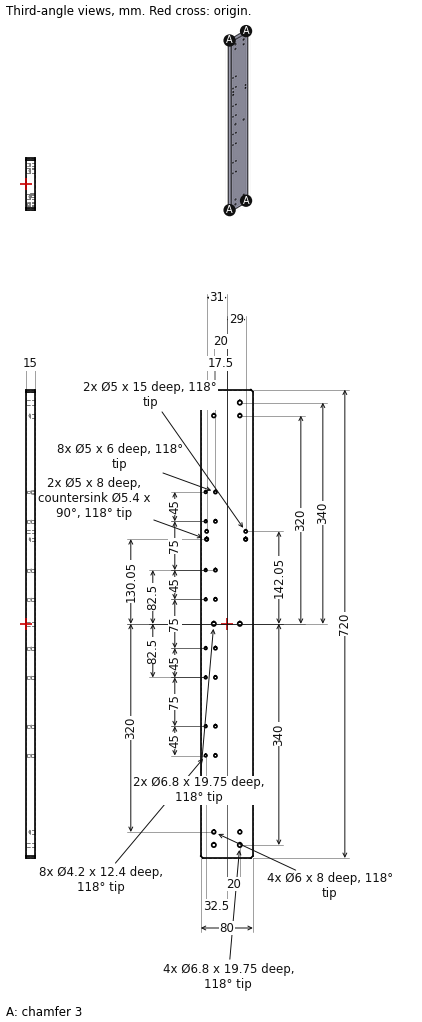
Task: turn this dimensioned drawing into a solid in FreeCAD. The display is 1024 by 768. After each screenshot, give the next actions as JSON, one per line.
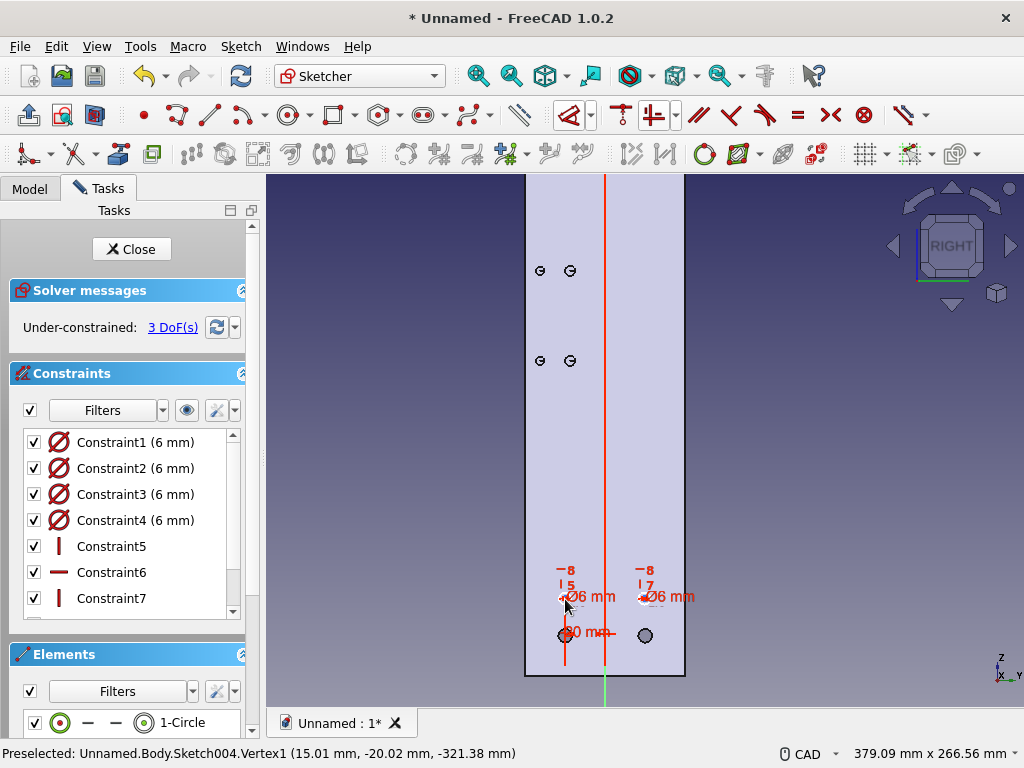
{"action": "scroll", "coordinate": [567, 599], "scroll_direction": "down", "scroll_amount": 7}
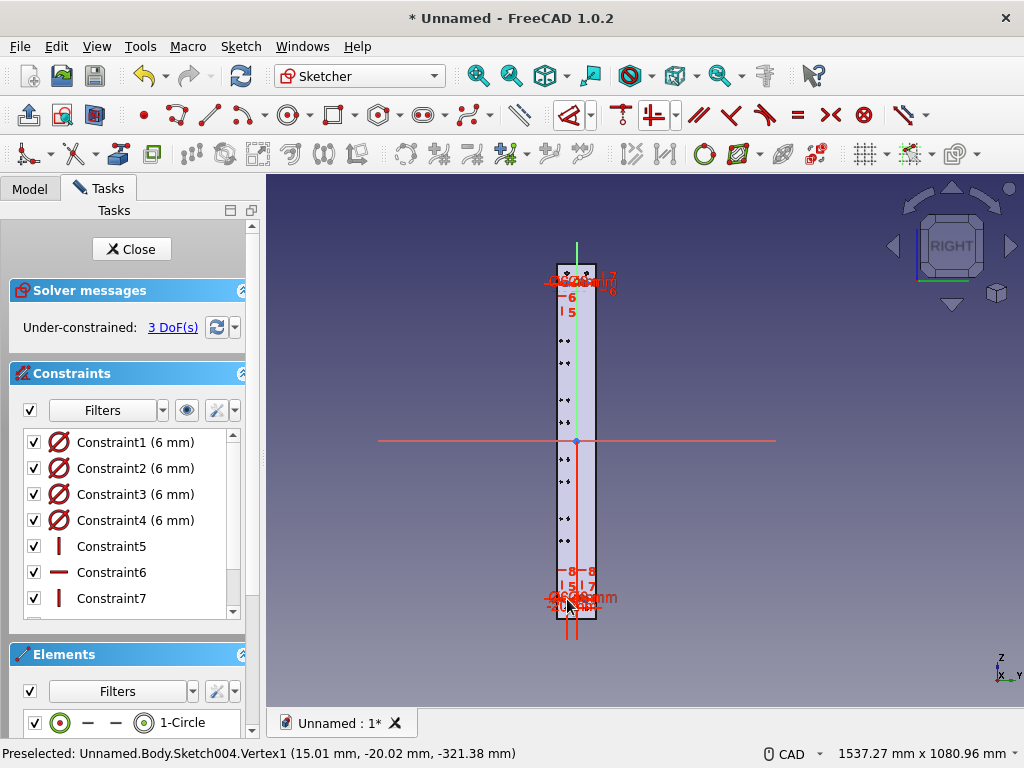
{"action": "scroll", "coordinate": [586, 284], "scroll_direction": "up", "scroll_amount": 7}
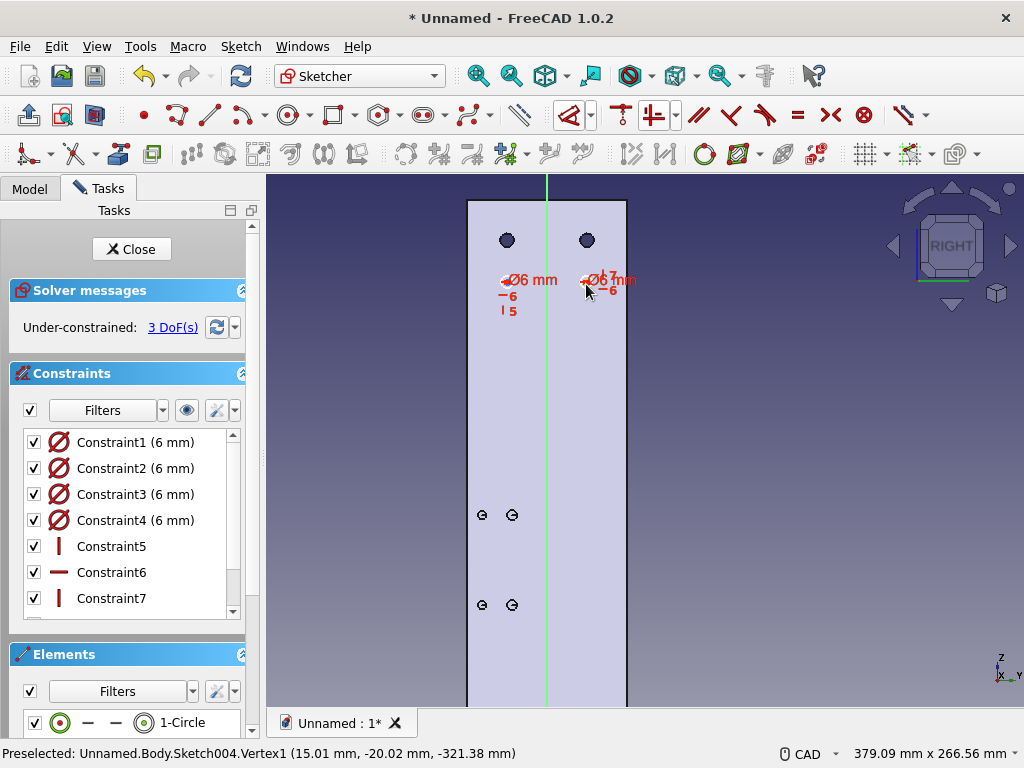
{"action": "left_click", "coordinate": [586, 282]}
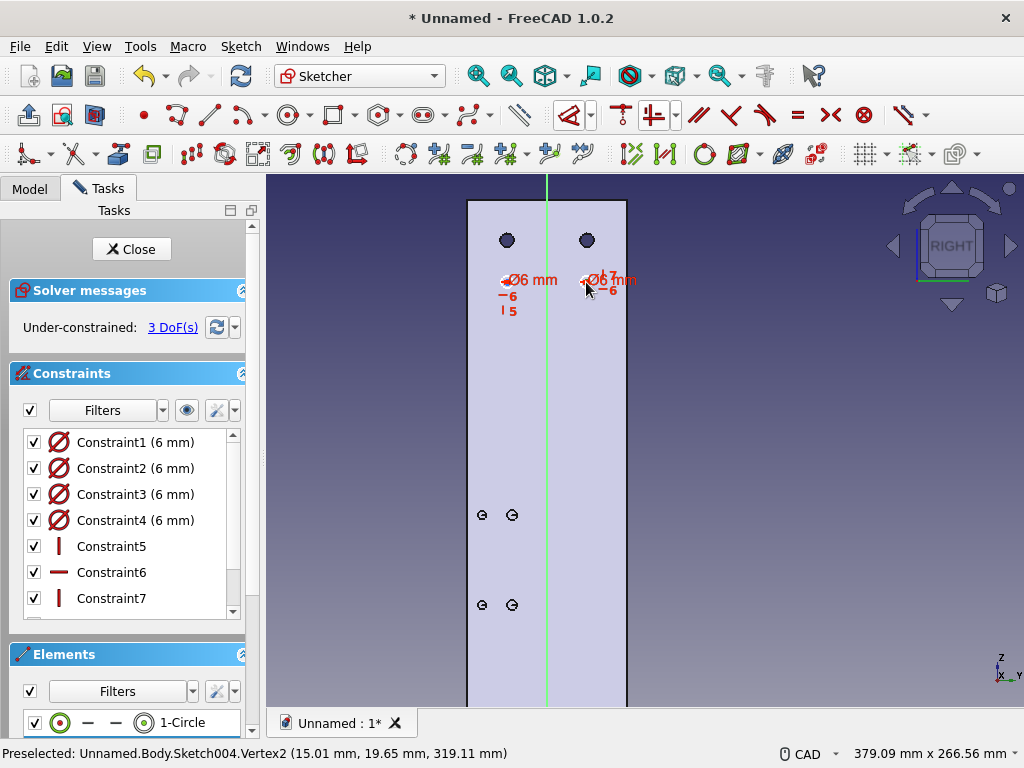
{"action": "left_click", "coordinate": [590, 116]}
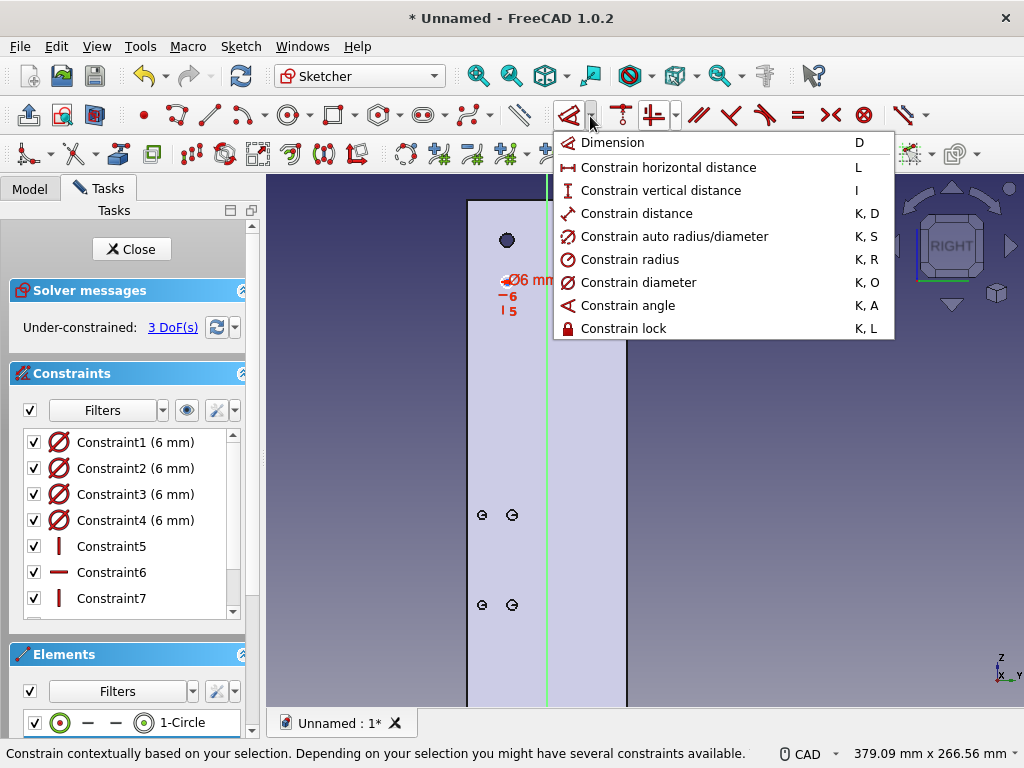
{"action": "left_click", "coordinate": [724, 168]}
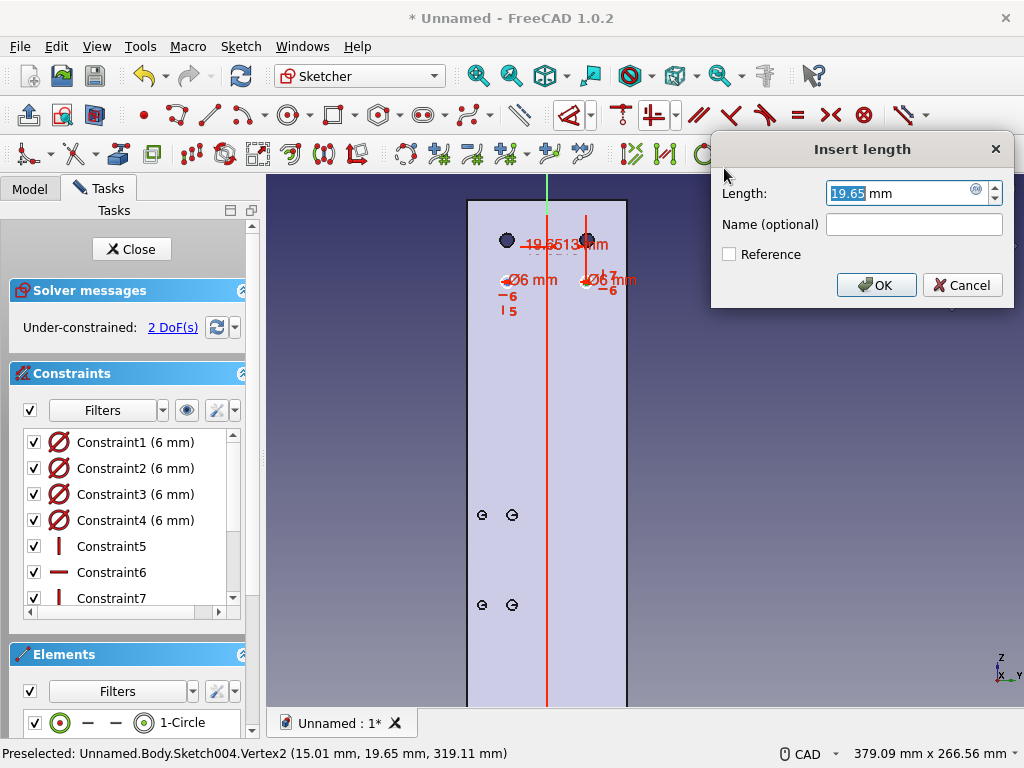
{"action": "type", "text": "20"}
{"action": "key", "text": "Return"}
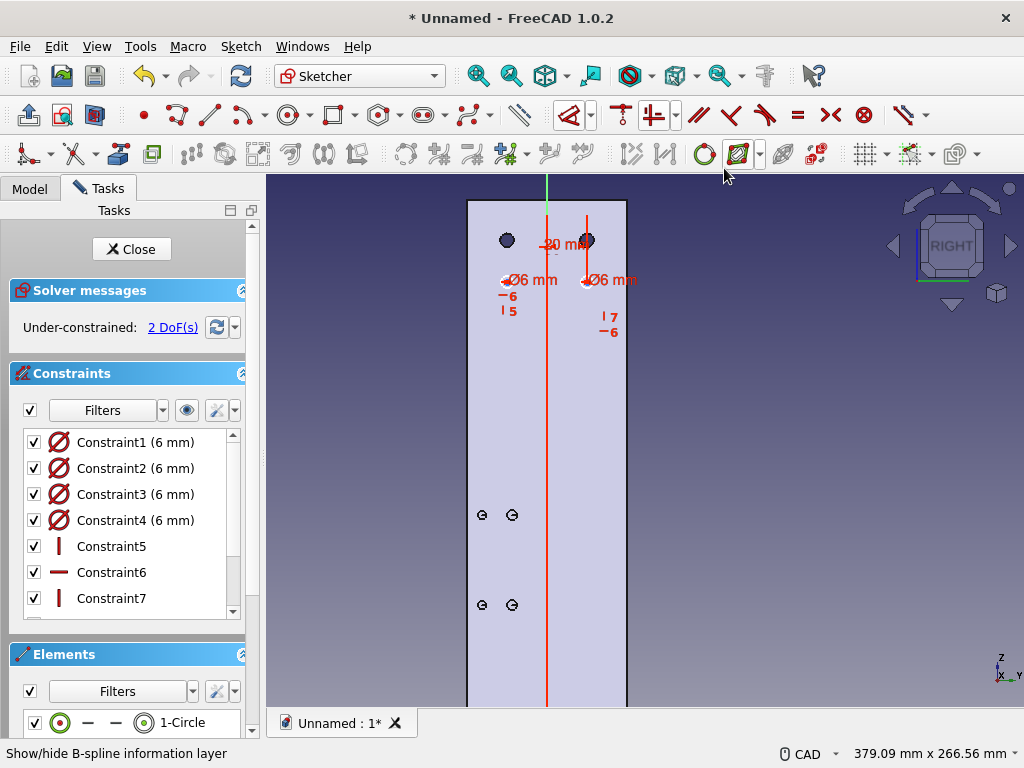
{"action": "scroll", "coordinate": [586, 284], "scroll_direction": "down", "scroll_amount": 7}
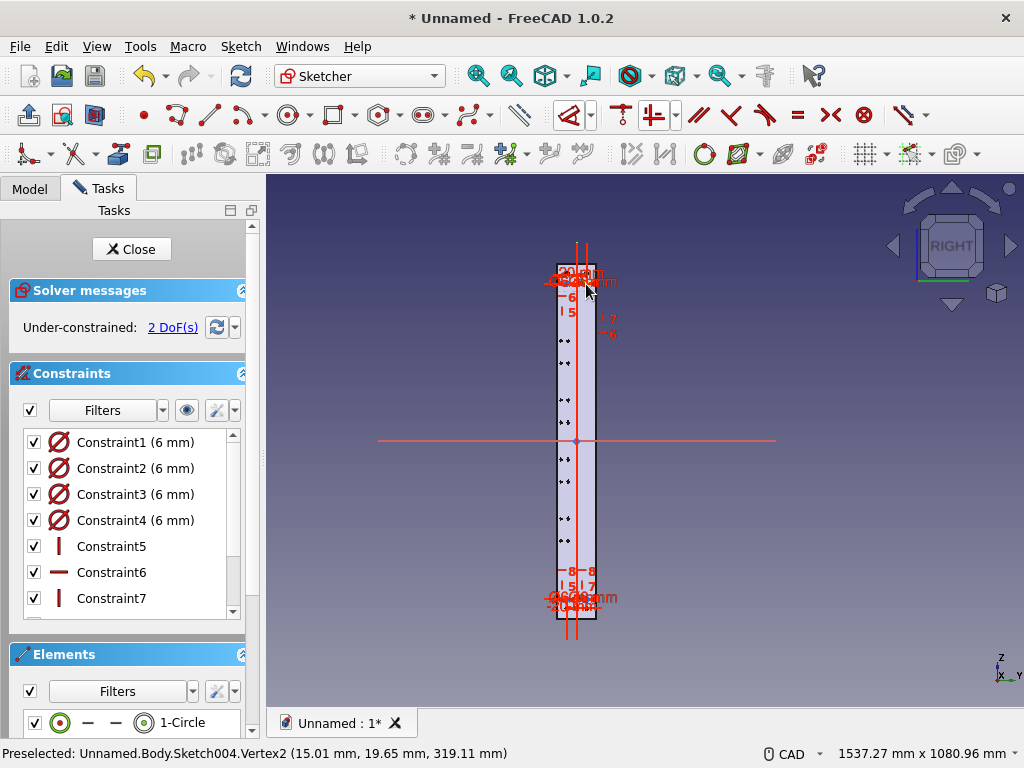
{"action": "left_click", "coordinate": [567, 599]}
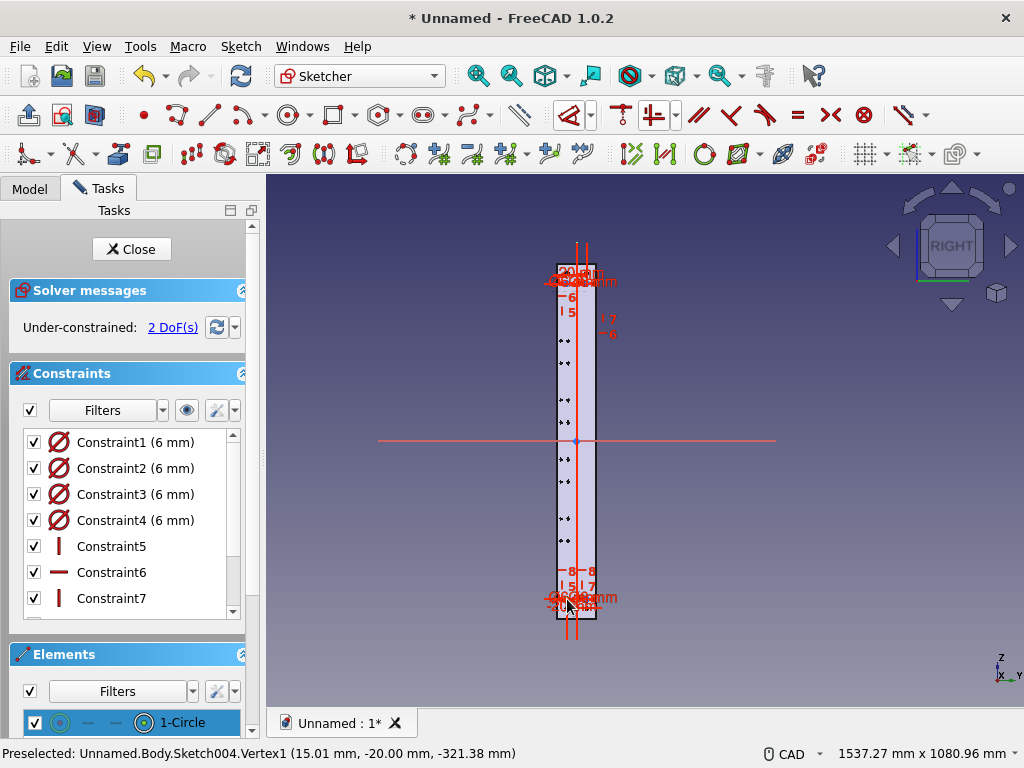
{"action": "left_click", "coordinate": [590, 116]}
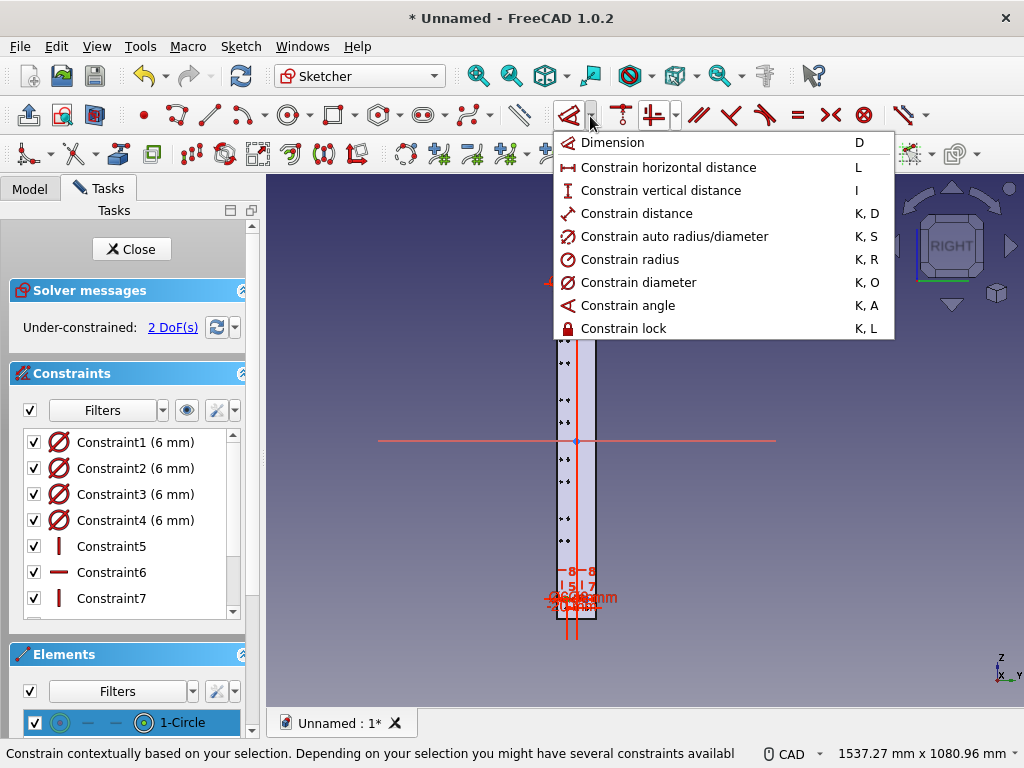
{"action": "left_click", "coordinate": [724, 190]}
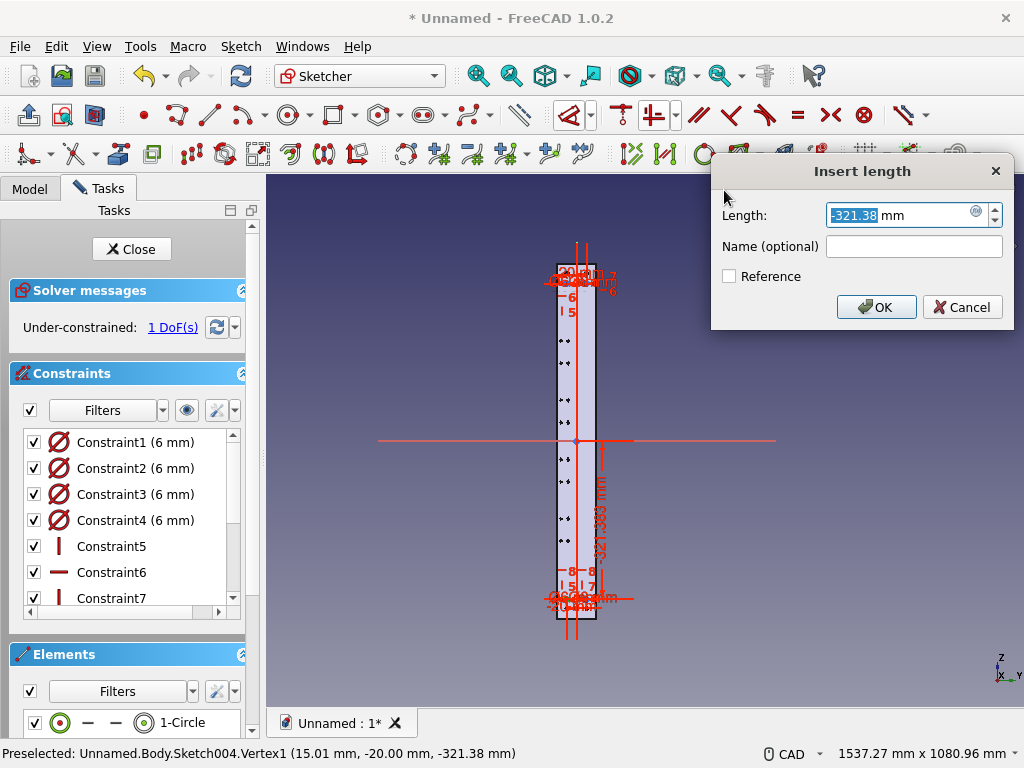
{"action": "type", "text": "-320"}
{"action": "key", "text": "Return"}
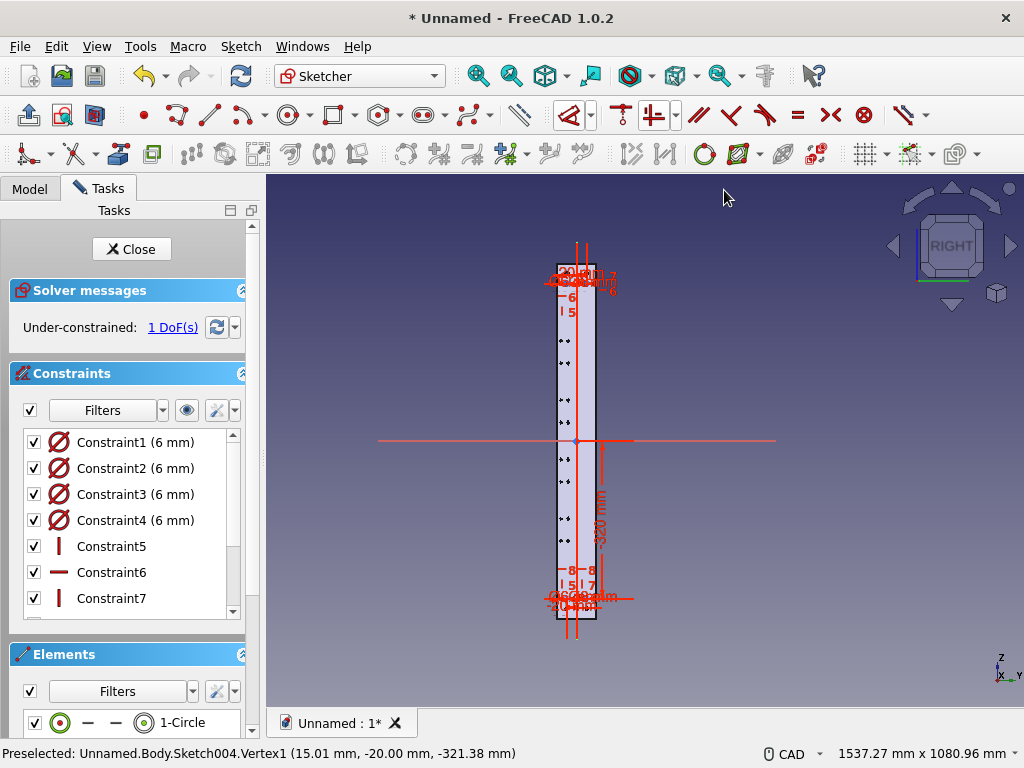
{"action": "left_click", "coordinate": [587, 284]}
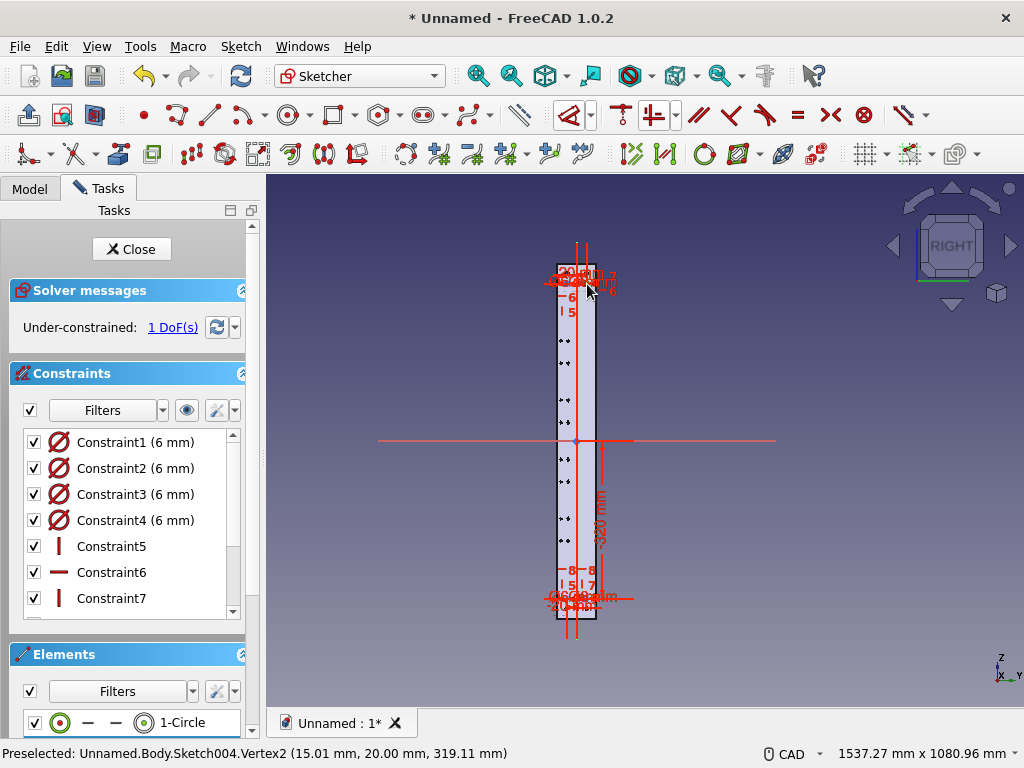
{"action": "left_click", "coordinate": [590, 116]}